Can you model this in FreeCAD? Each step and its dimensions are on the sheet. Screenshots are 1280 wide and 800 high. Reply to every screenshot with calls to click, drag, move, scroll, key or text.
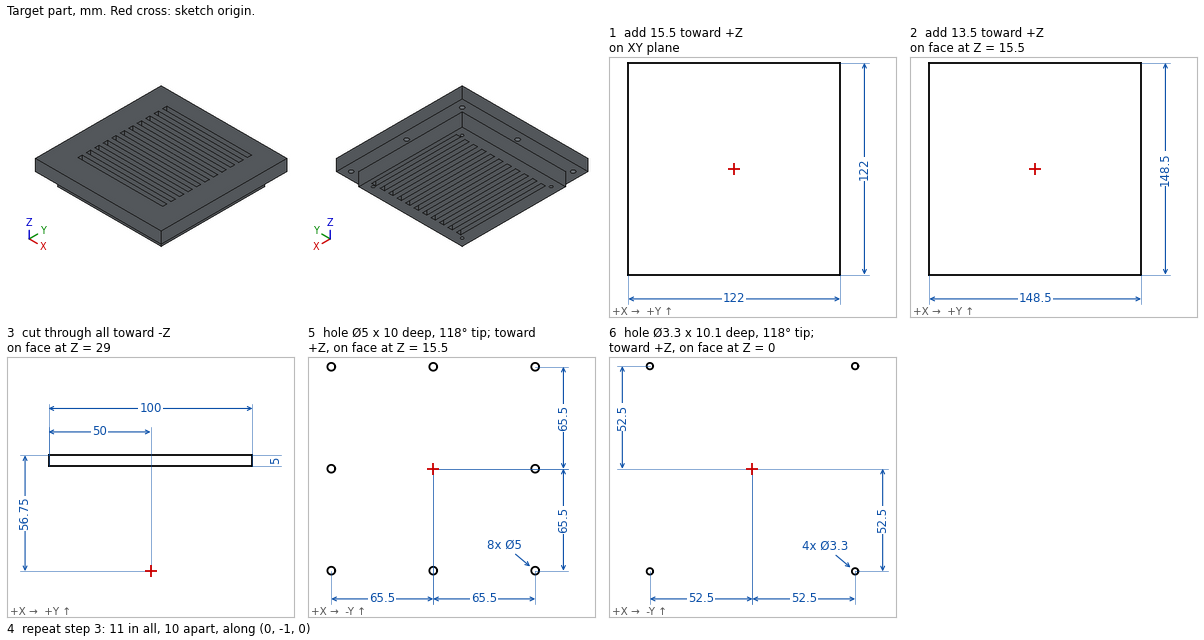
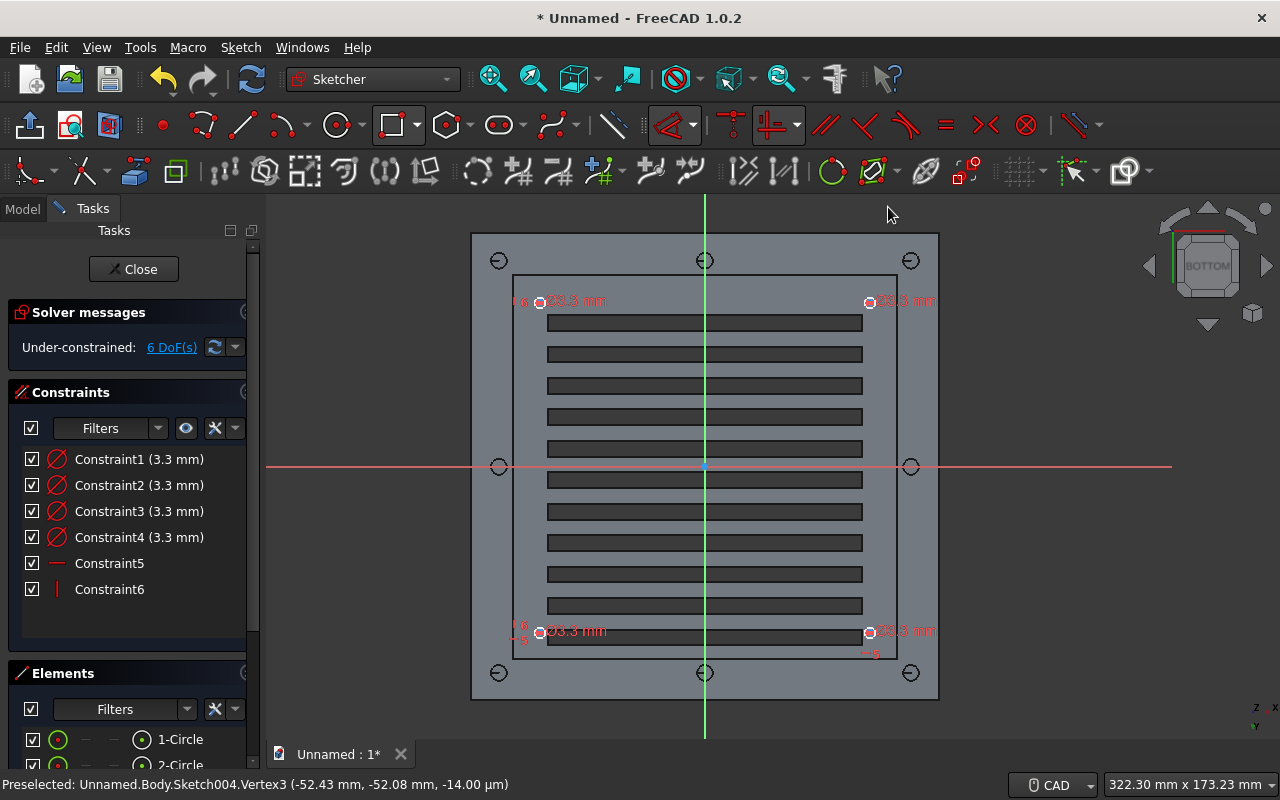
click(870, 633)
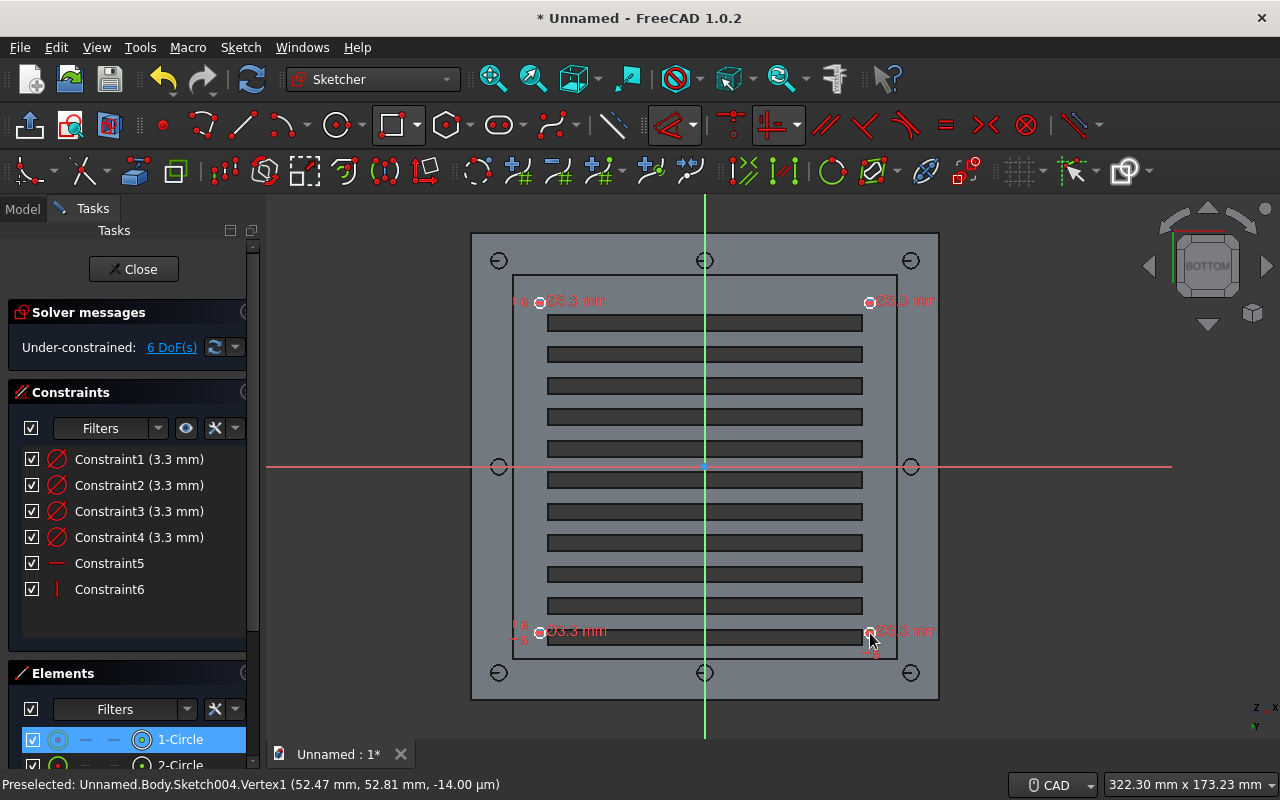
click(870, 303)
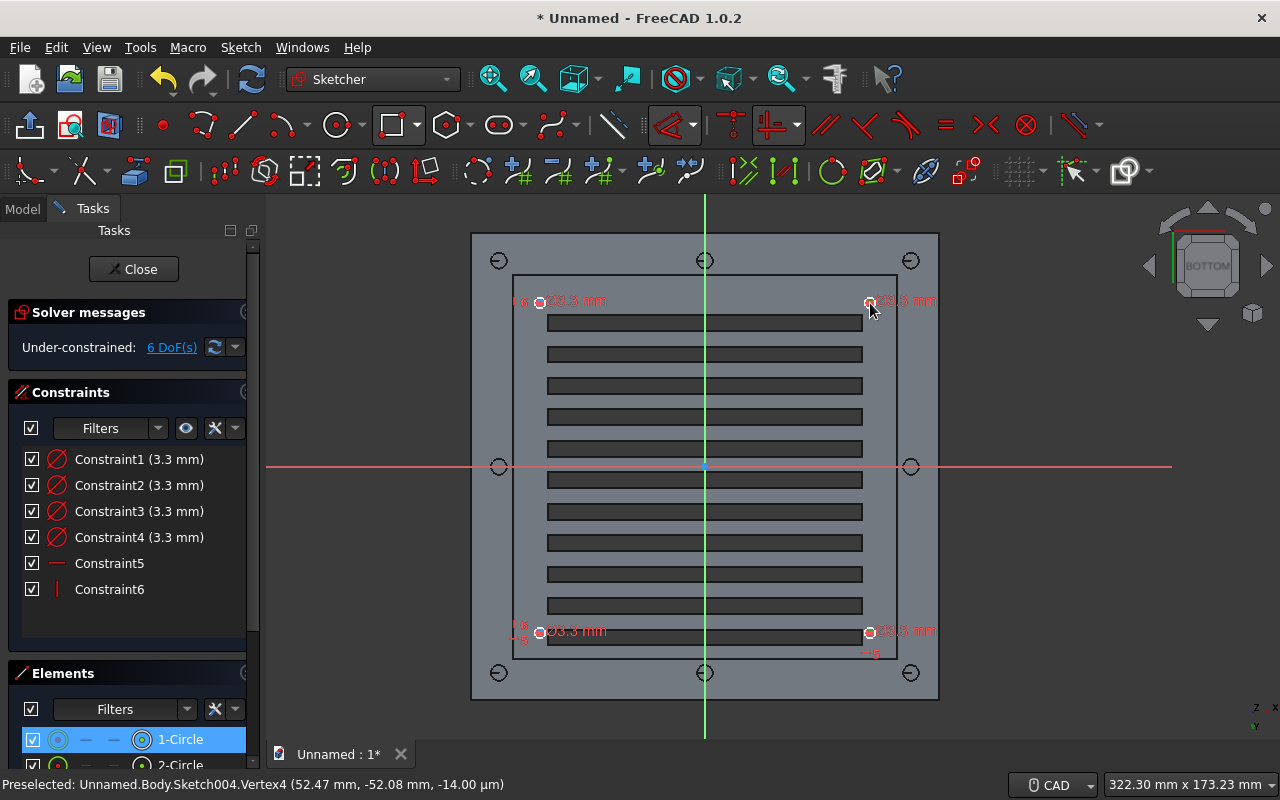
click(800, 126)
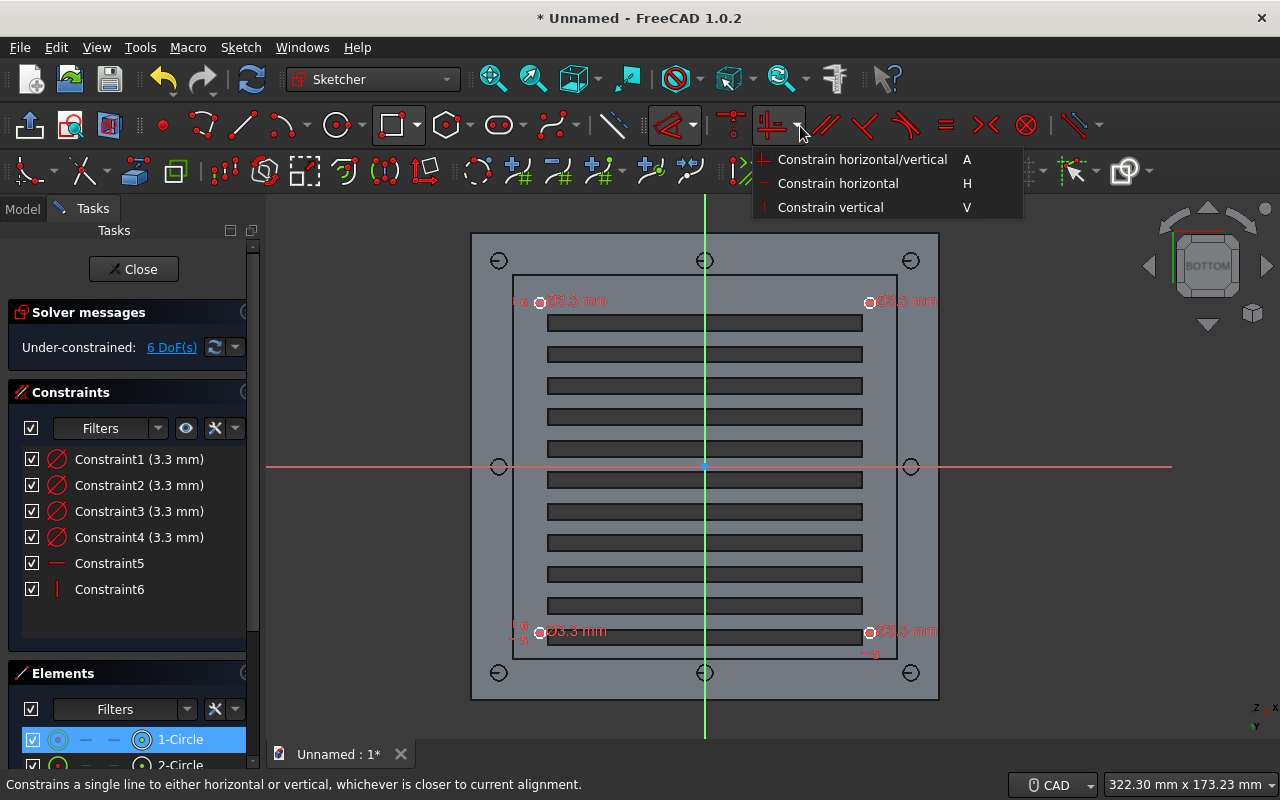
click(888, 207)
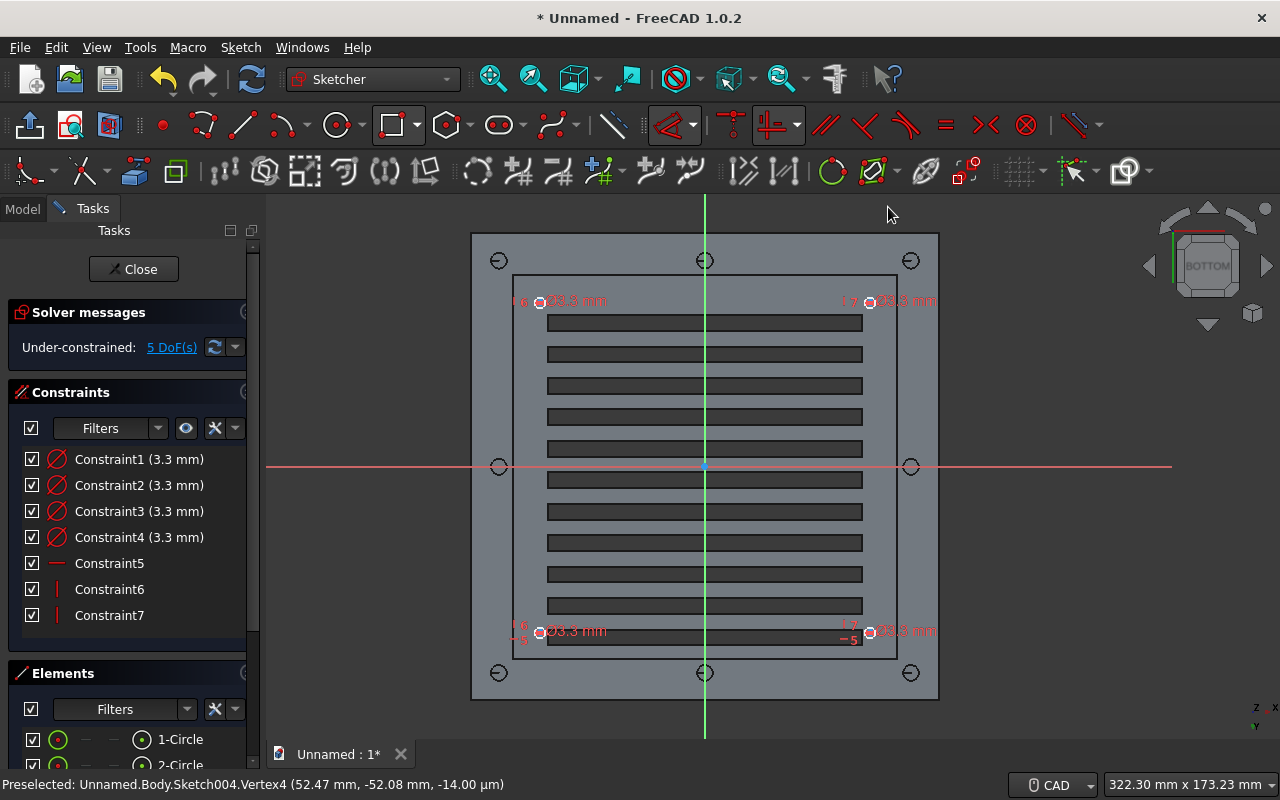
click(540, 303)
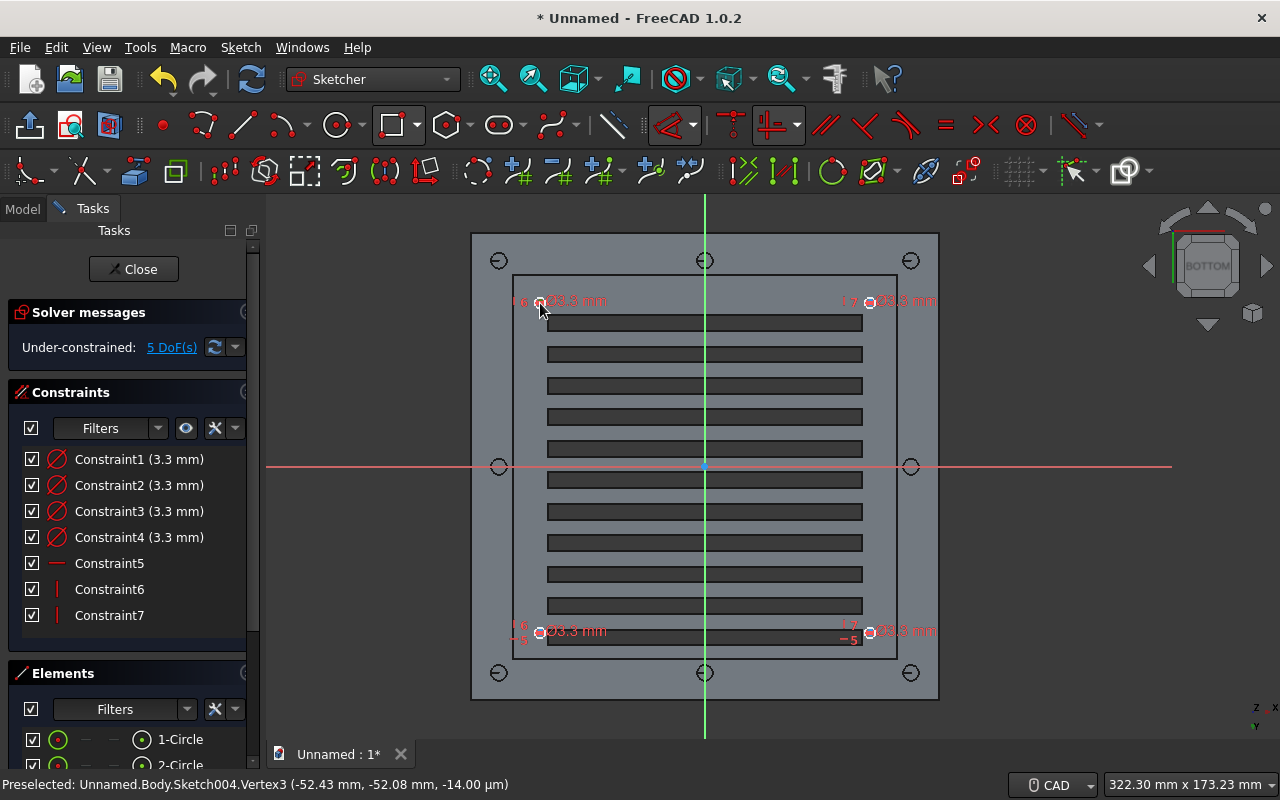
click(870, 303)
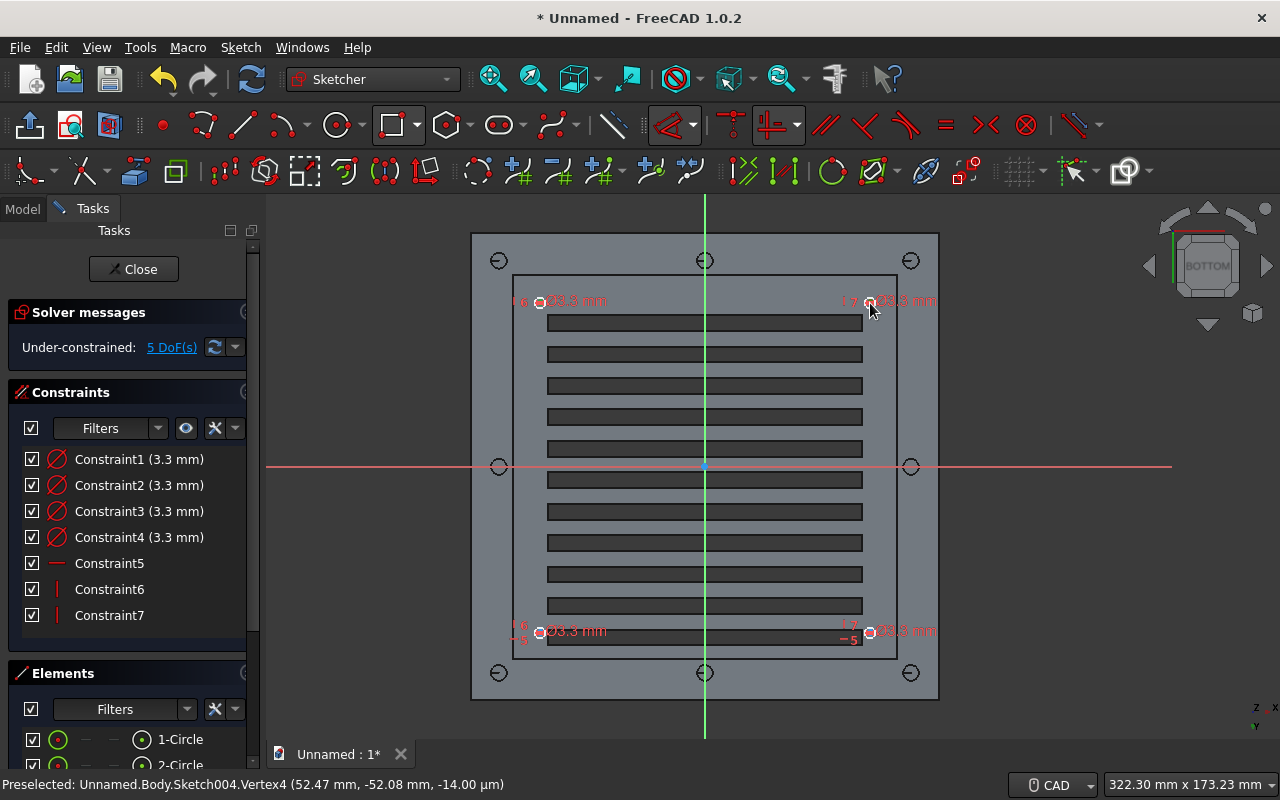
click(800, 126)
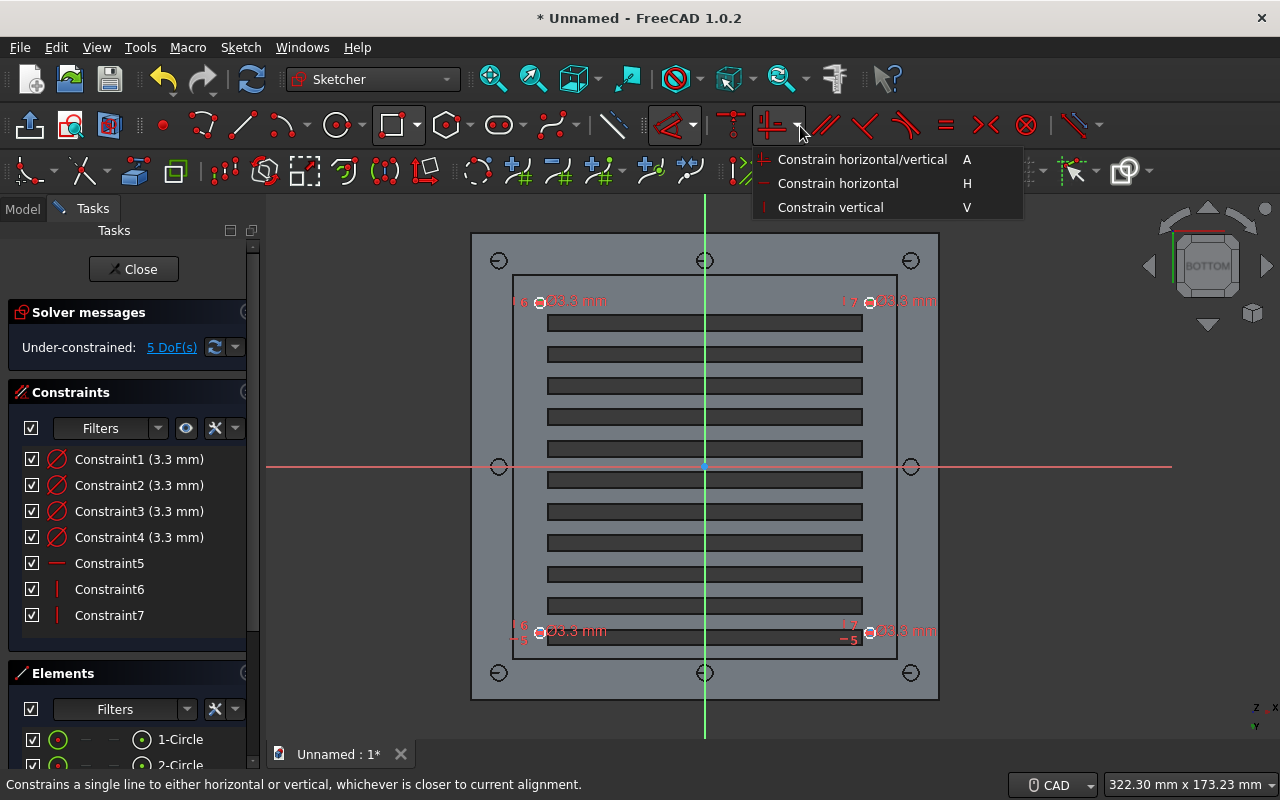
click(888, 183)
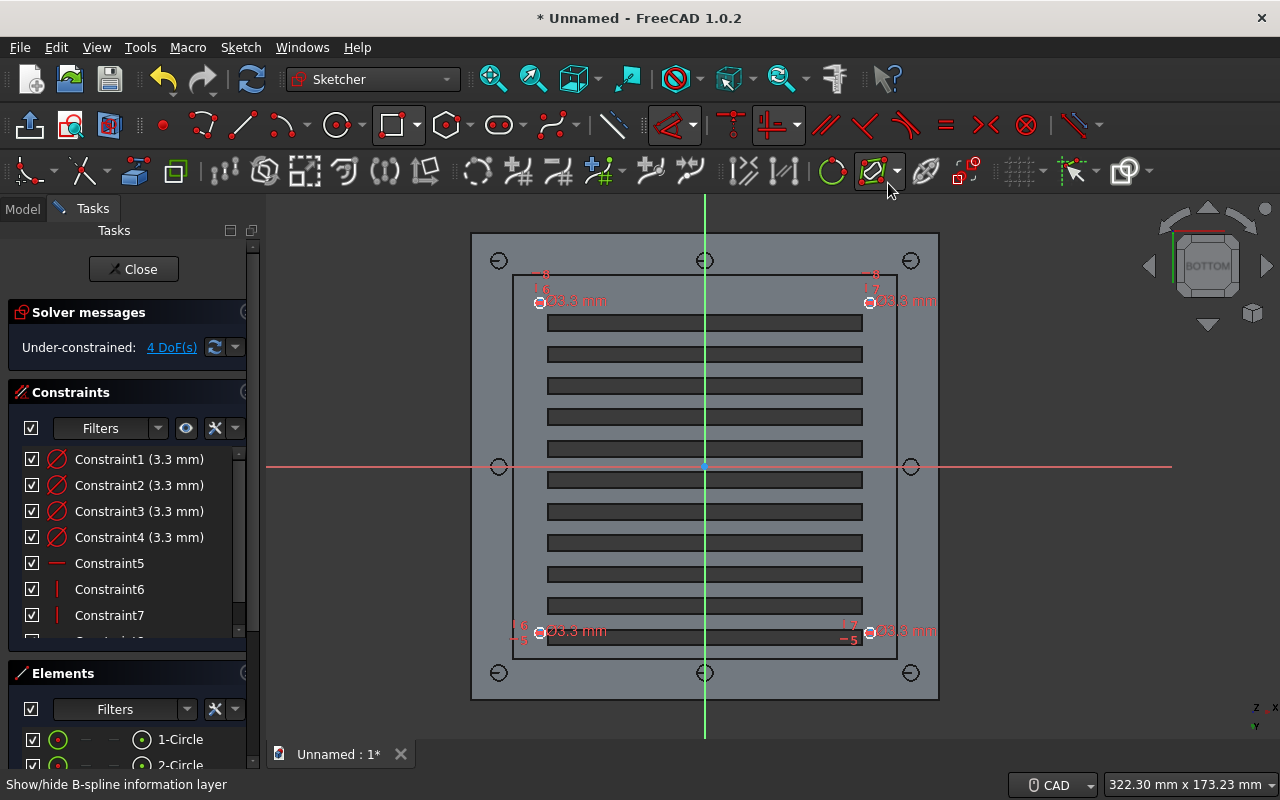
click(870, 633)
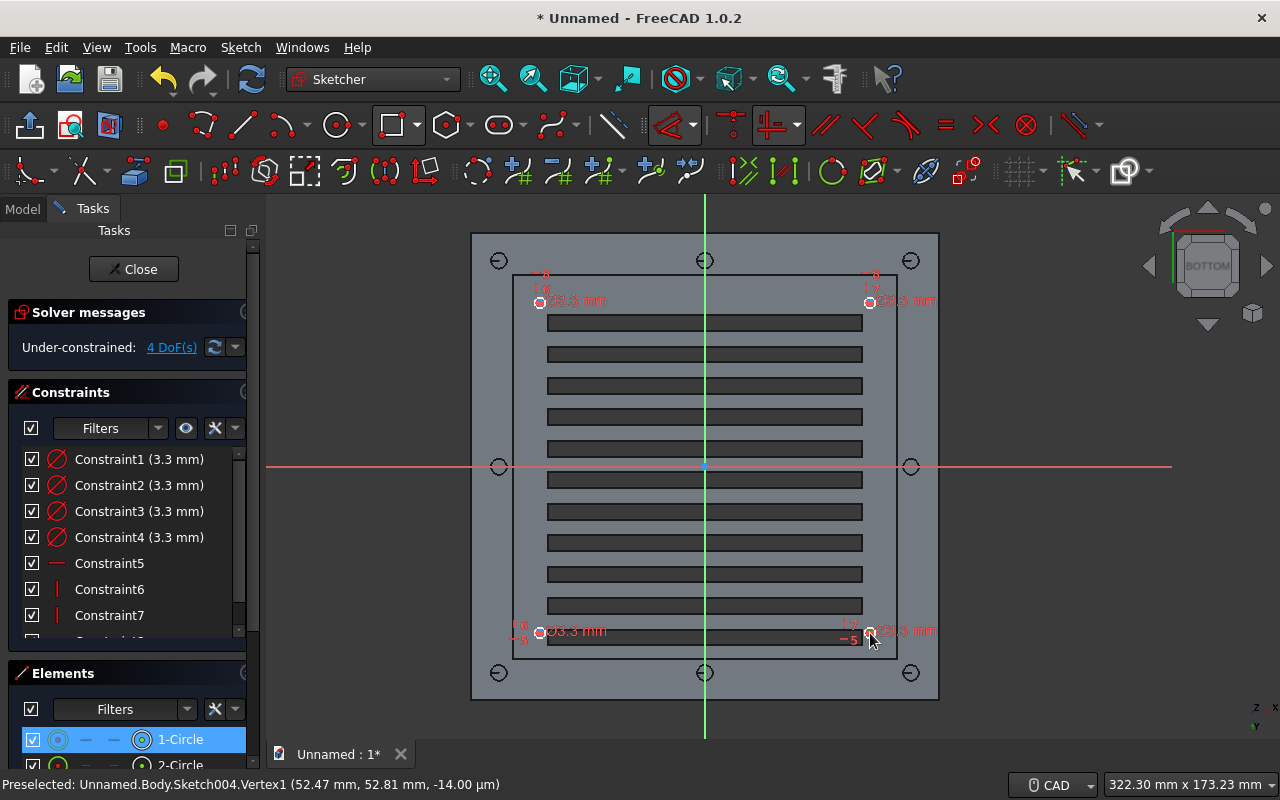
click(696, 126)